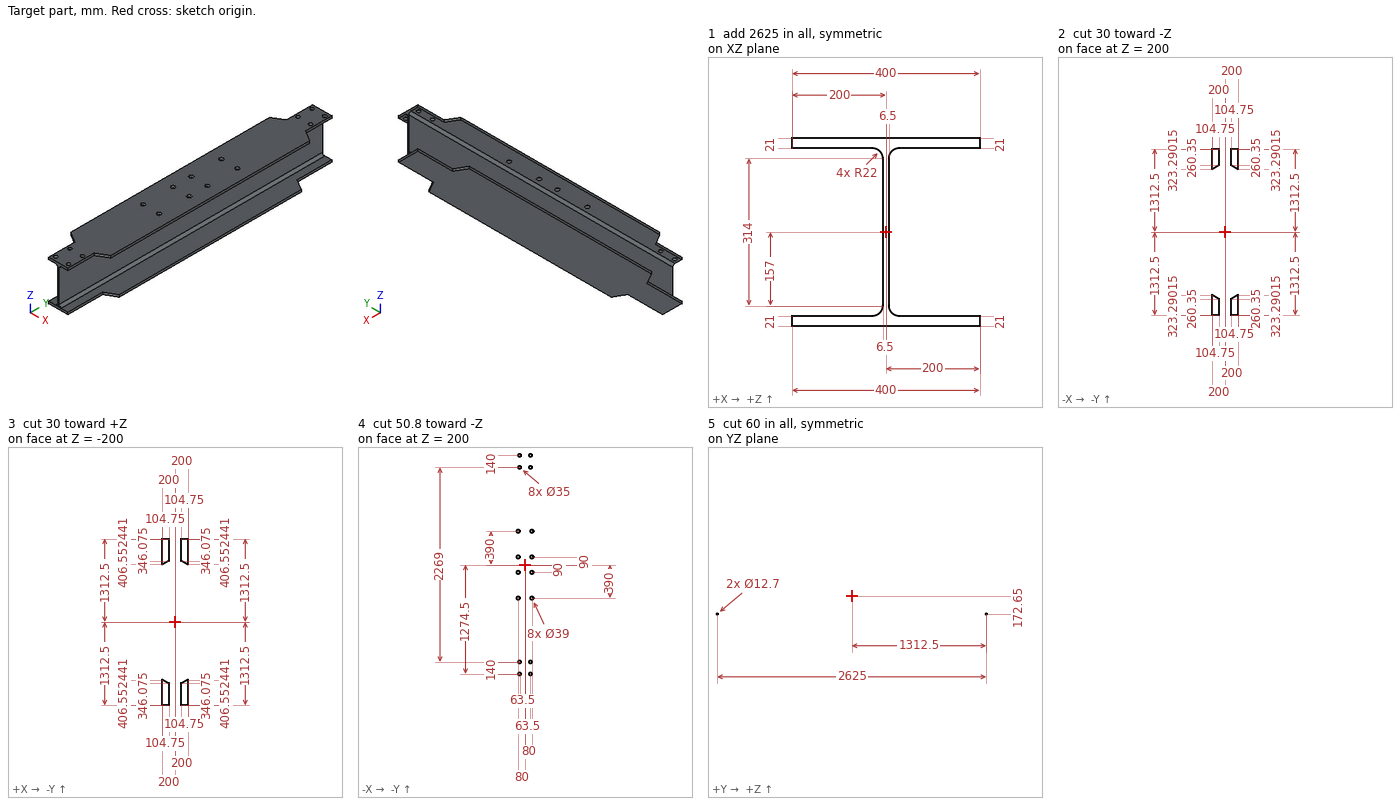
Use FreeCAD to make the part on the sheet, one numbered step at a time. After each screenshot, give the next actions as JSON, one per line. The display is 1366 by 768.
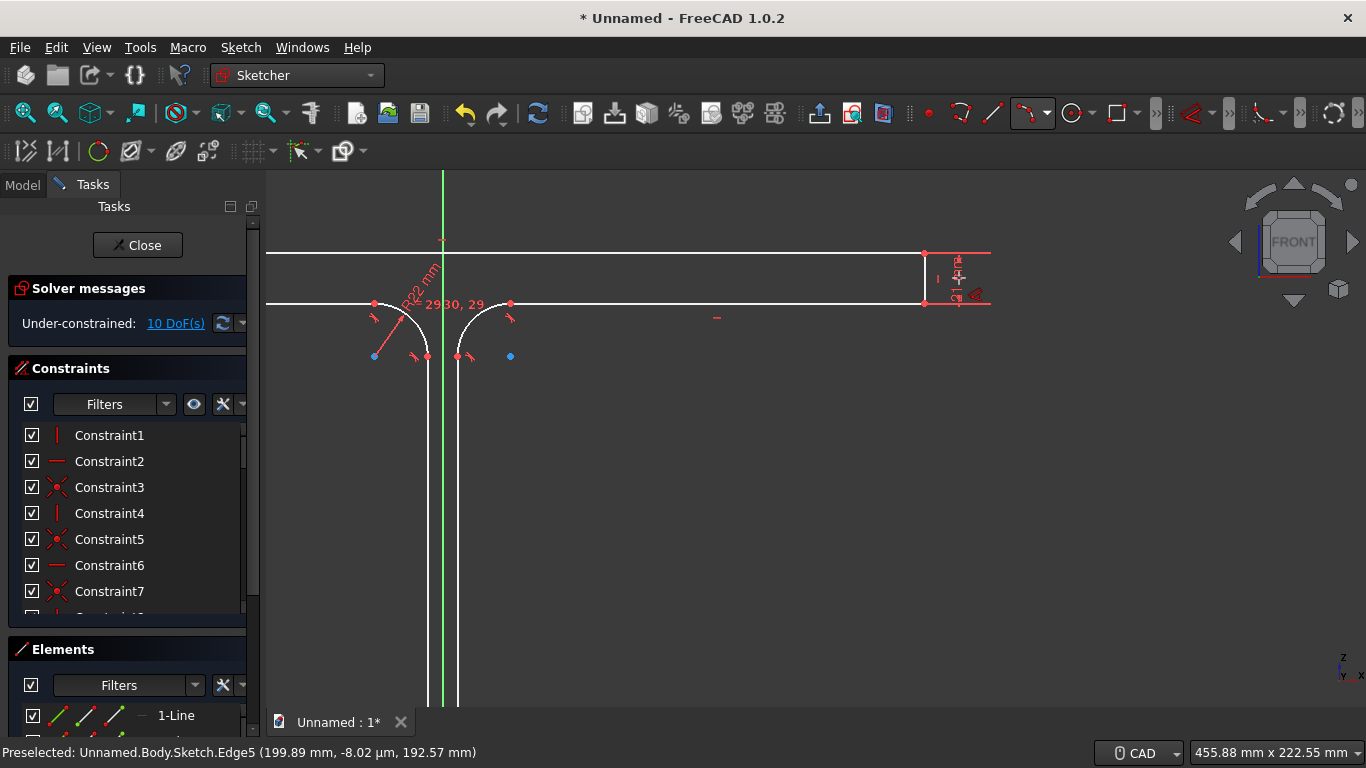
{"action": "scroll", "coordinate": [925, 267], "scroll_direction": "down", "scroll_amount": 5}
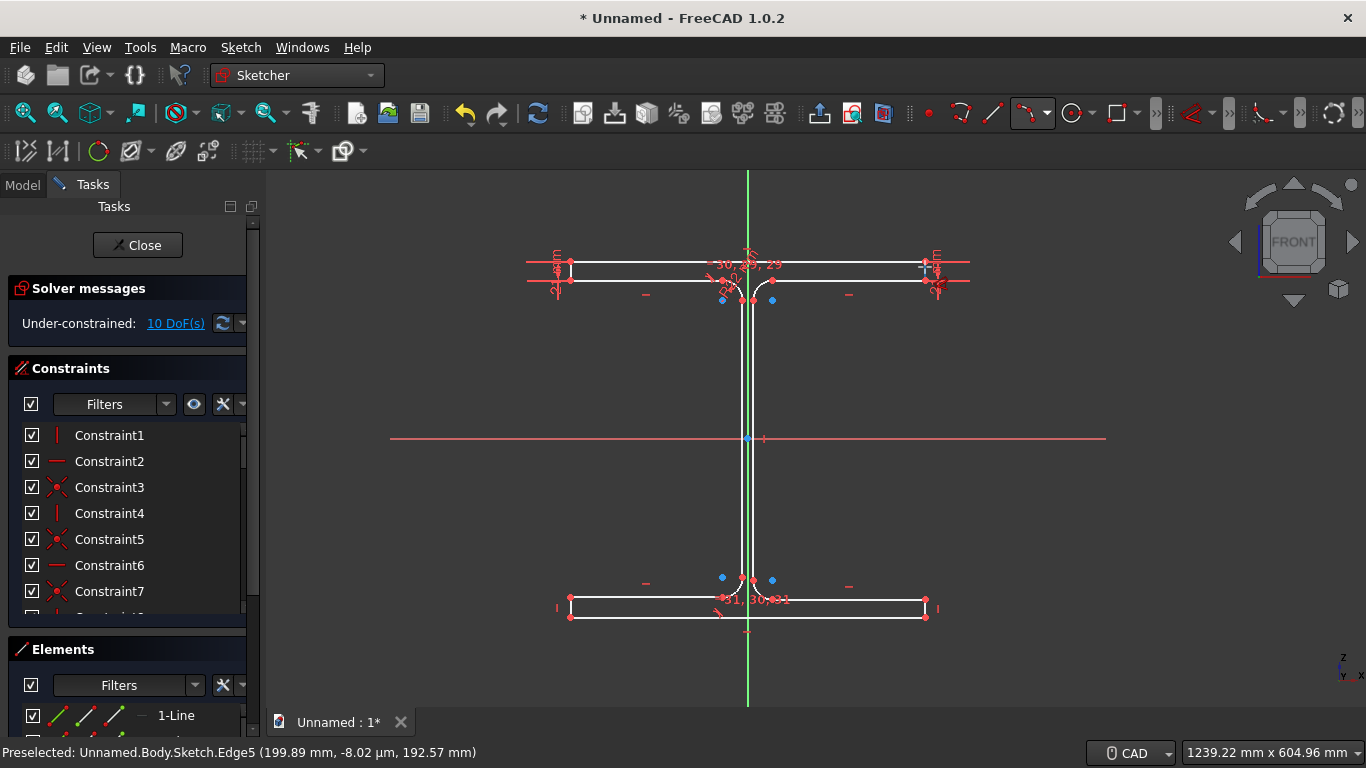
{"action": "scroll", "coordinate": [925, 605], "scroll_direction": "up", "scroll_amount": 5}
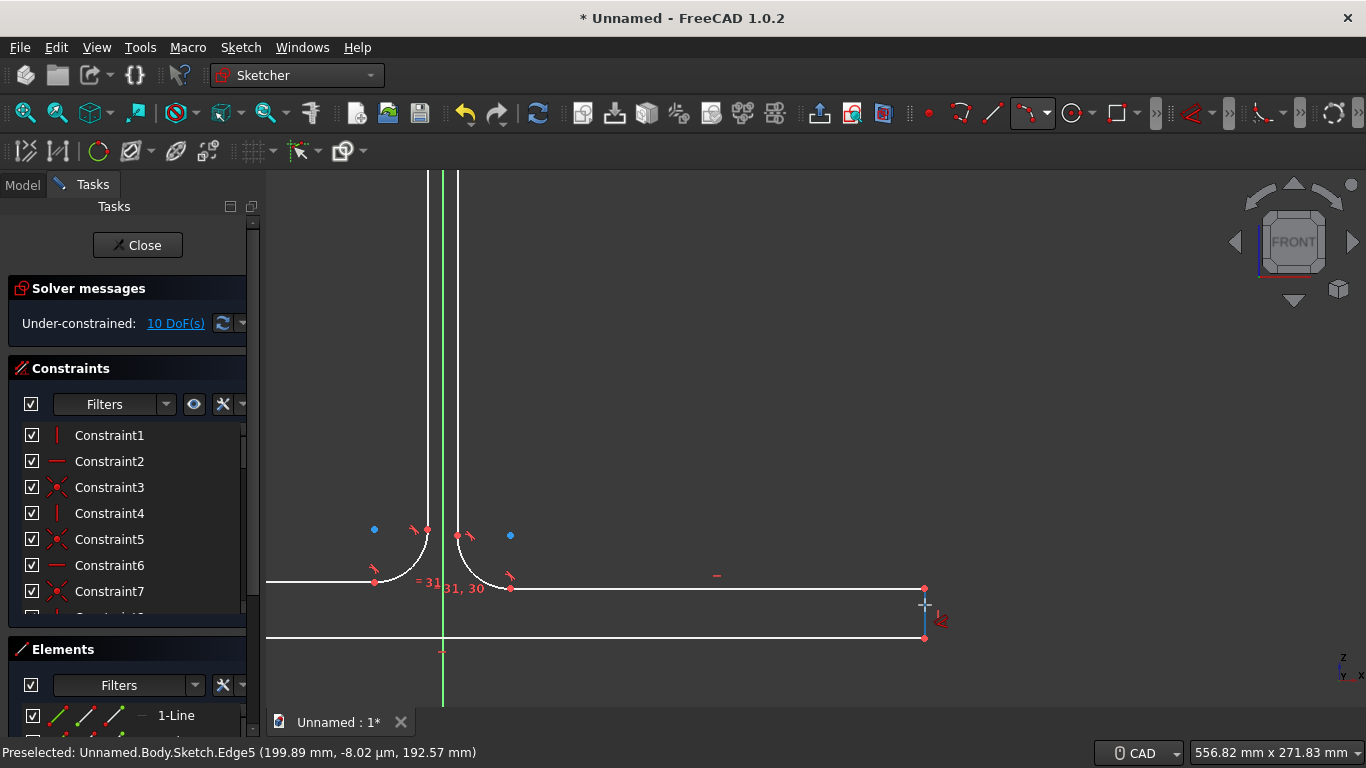
{"action": "left_click", "coordinate": [925, 604]}
{"action": "left_click", "coordinate": [959, 614]}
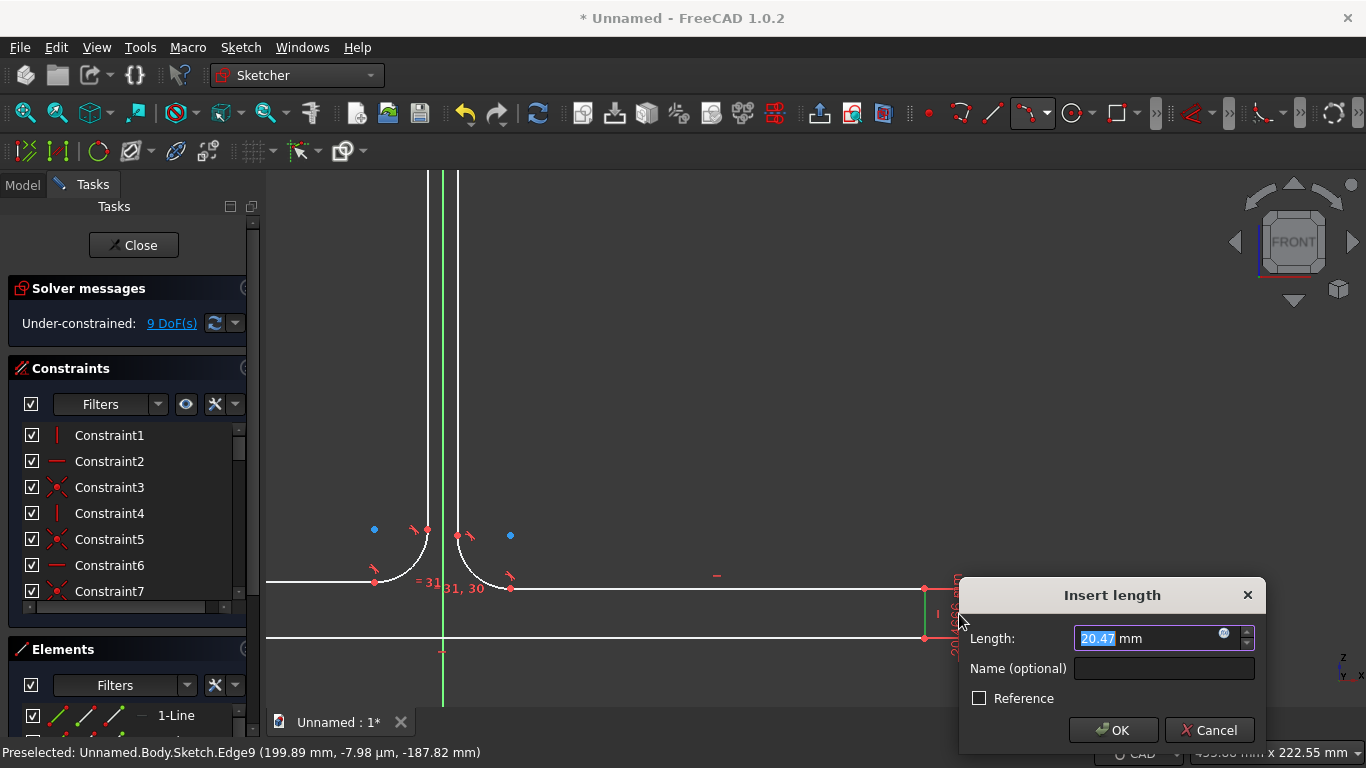
{"action": "type", "text": "21"}
{"action": "key", "text": "Return"}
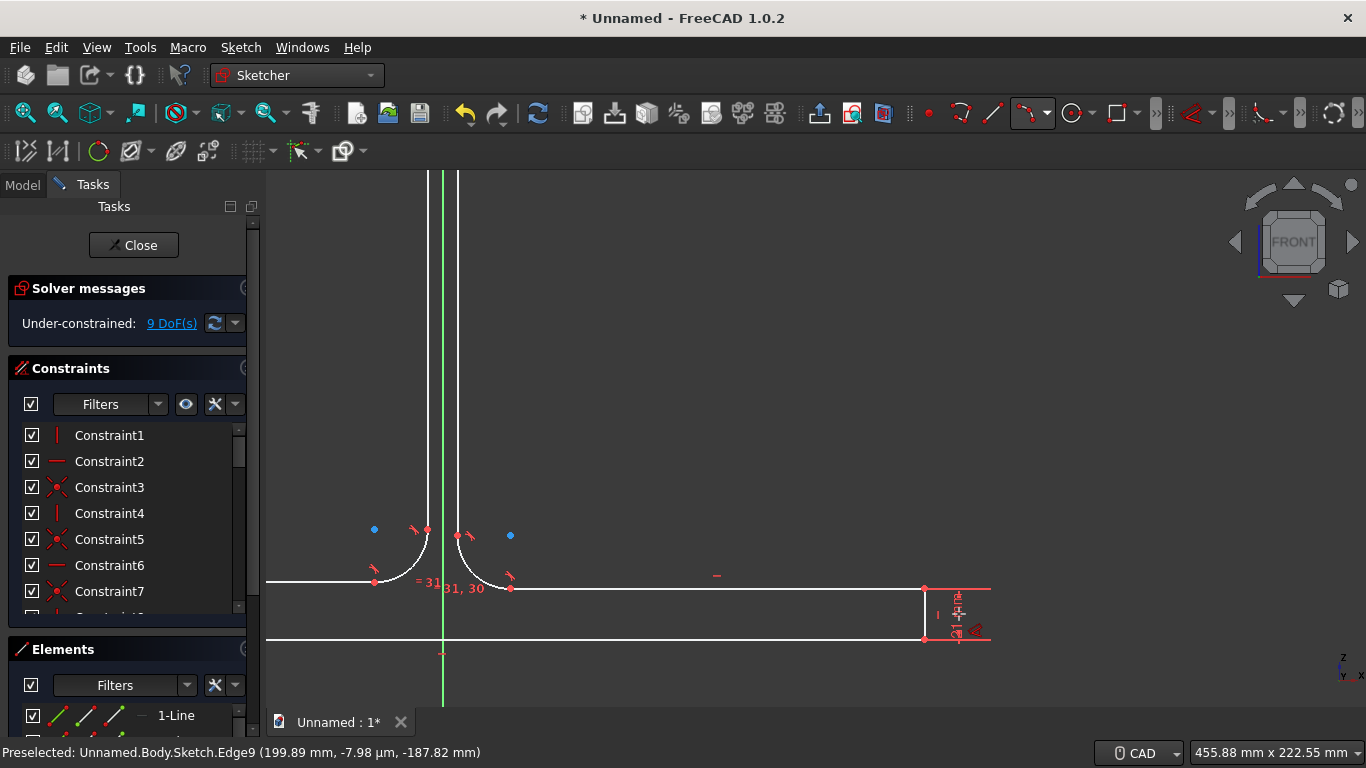
{"action": "scroll", "coordinate": [925, 605], "scroll_direction": "down", "scroll_amount": 5}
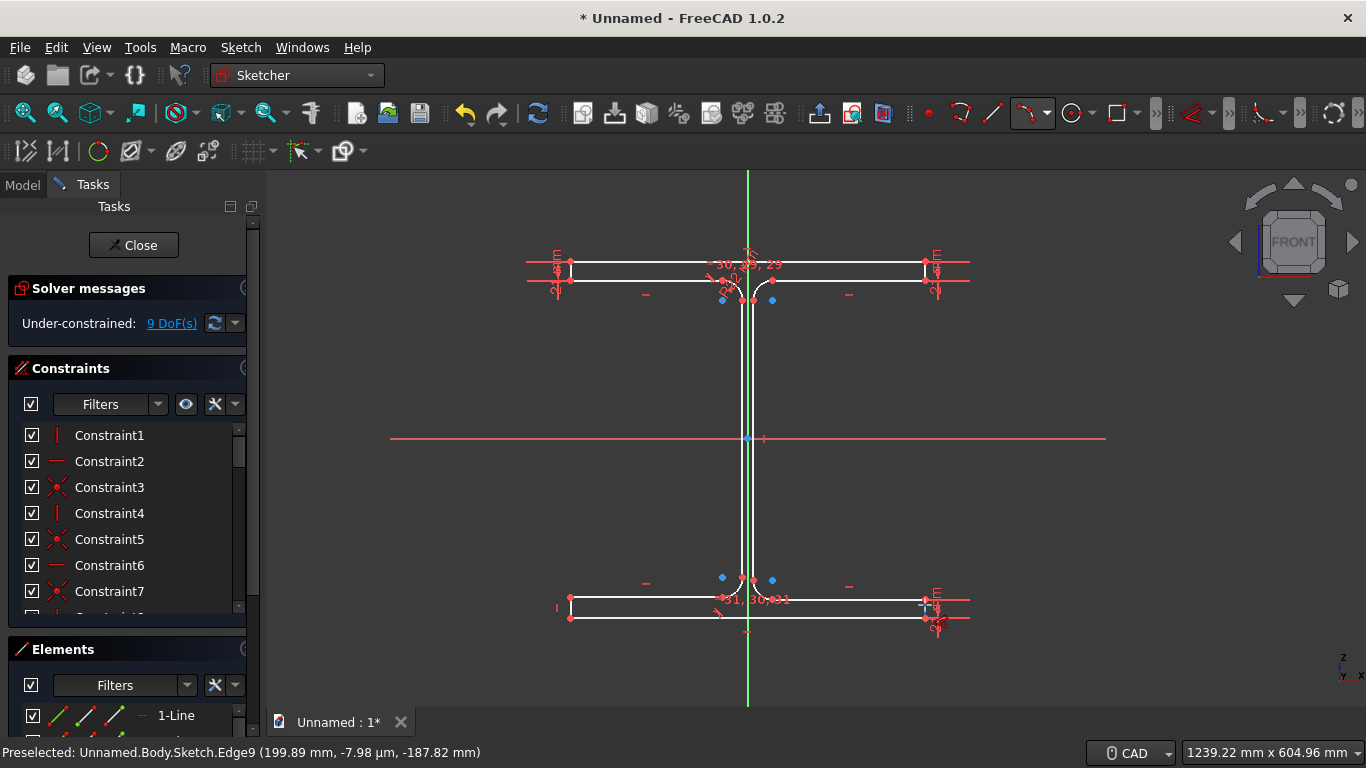
{"action": "scroll", "coordinate": [571, 612], "scroll_direction": "up", "scroll_amount": 4}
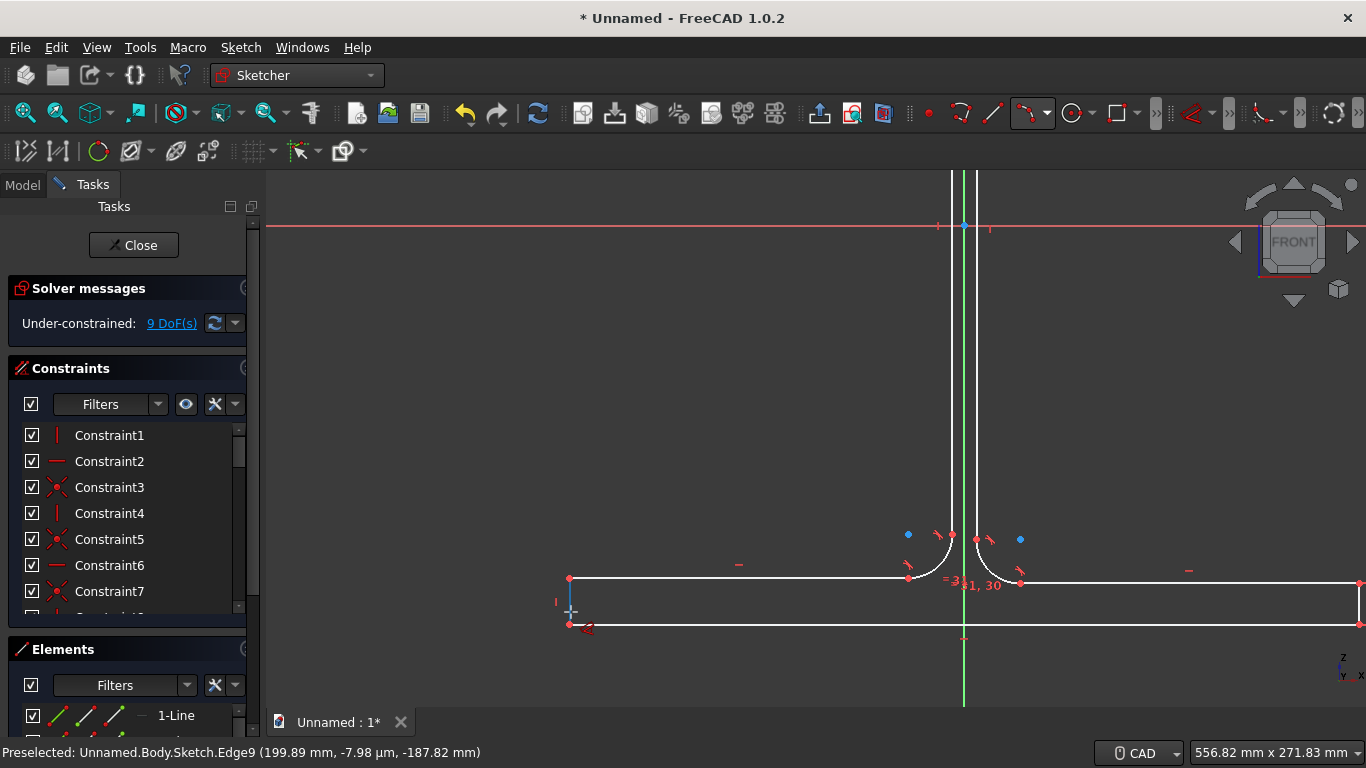
{"action": "left_click", "coordinate": [570, 611]}
{"action": "left_click", "coordinate": [536, 601]}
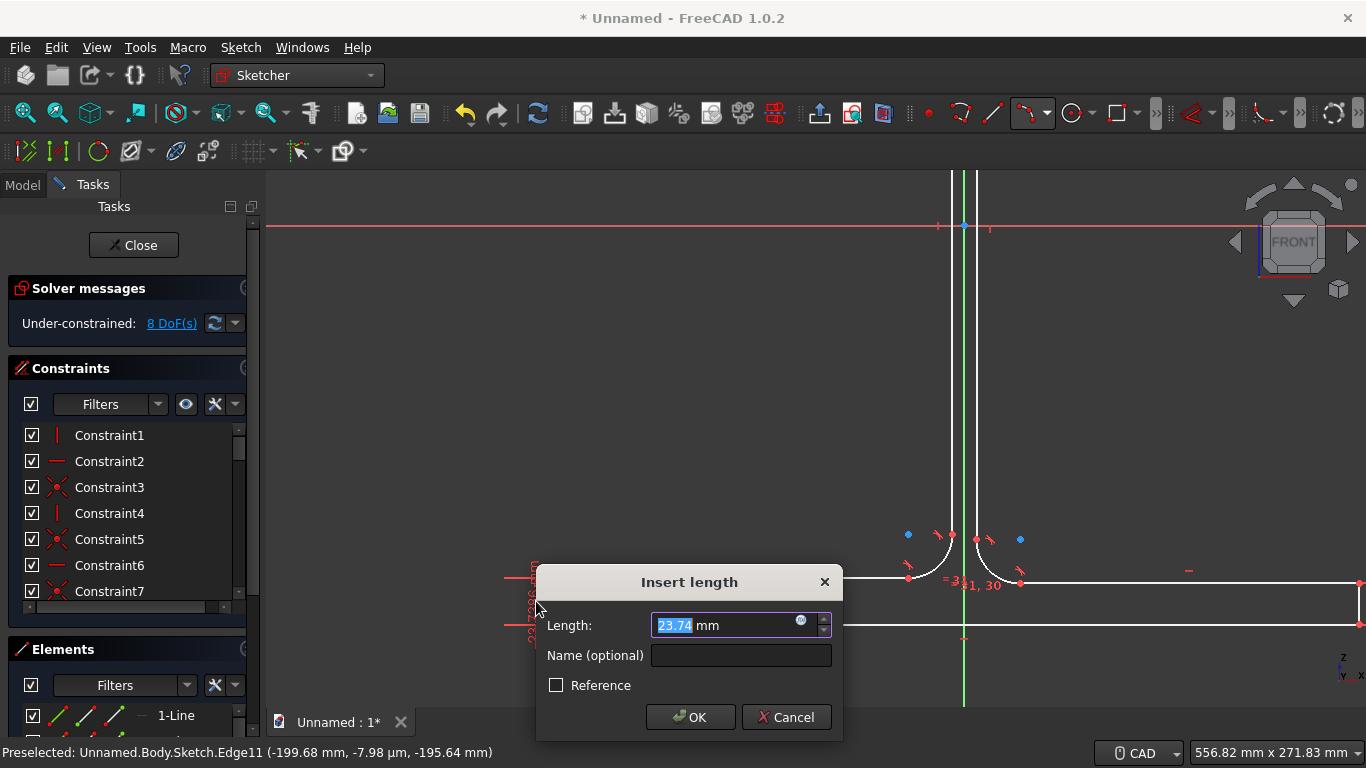
{"action": "type", "text": "21"}
{"action": "key", "text": "Return"}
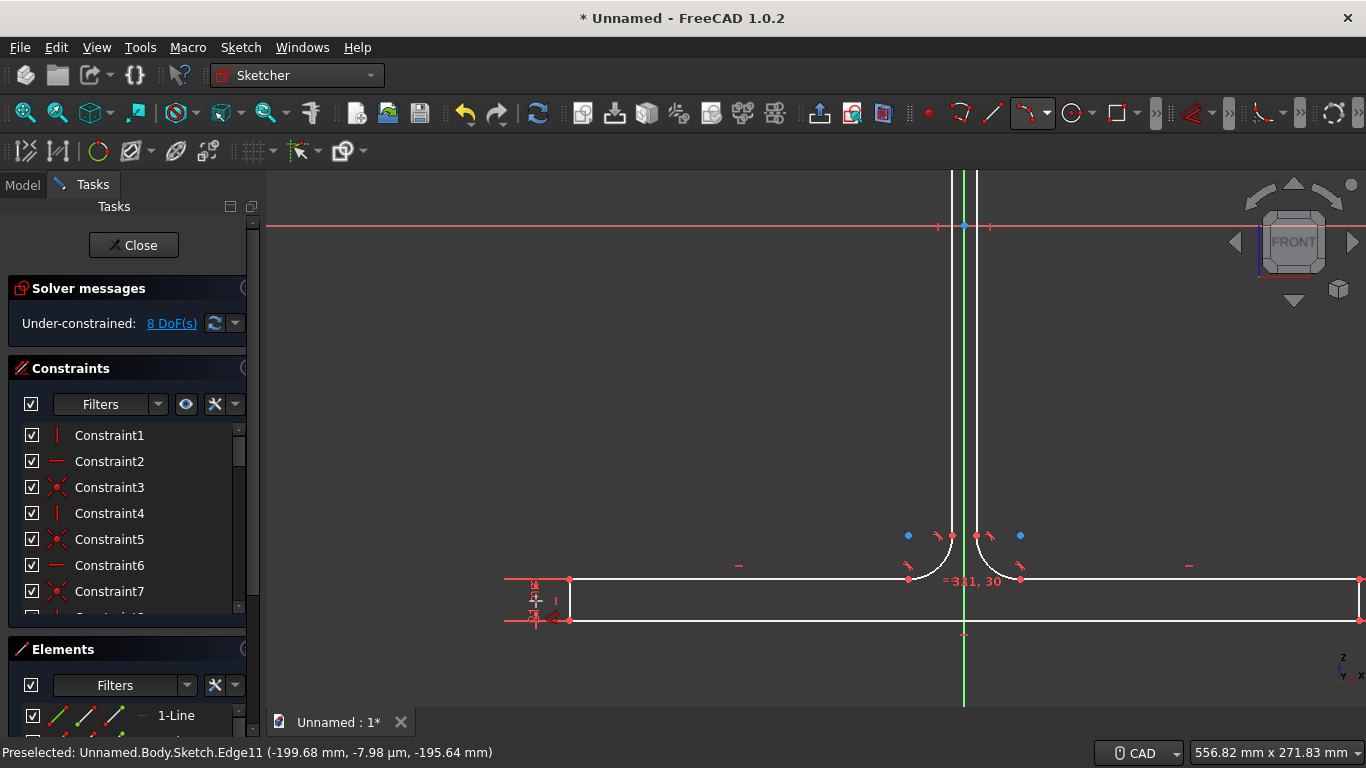
{"action": "left_click", "coordinate": [952, 350]}
{"action": "left_click", "coordinate": [918, 367]}